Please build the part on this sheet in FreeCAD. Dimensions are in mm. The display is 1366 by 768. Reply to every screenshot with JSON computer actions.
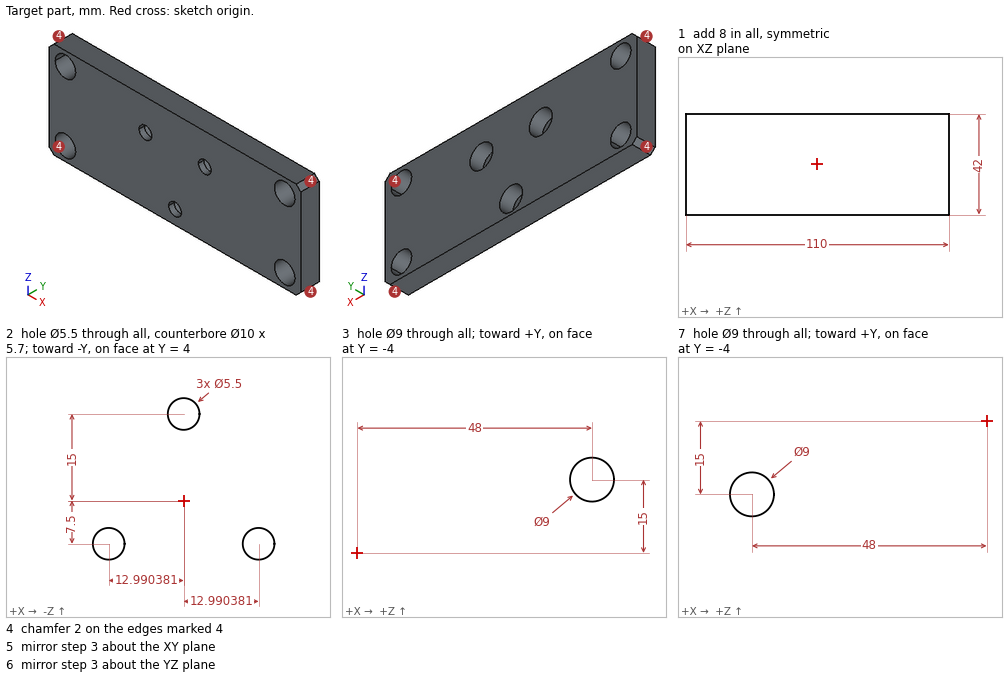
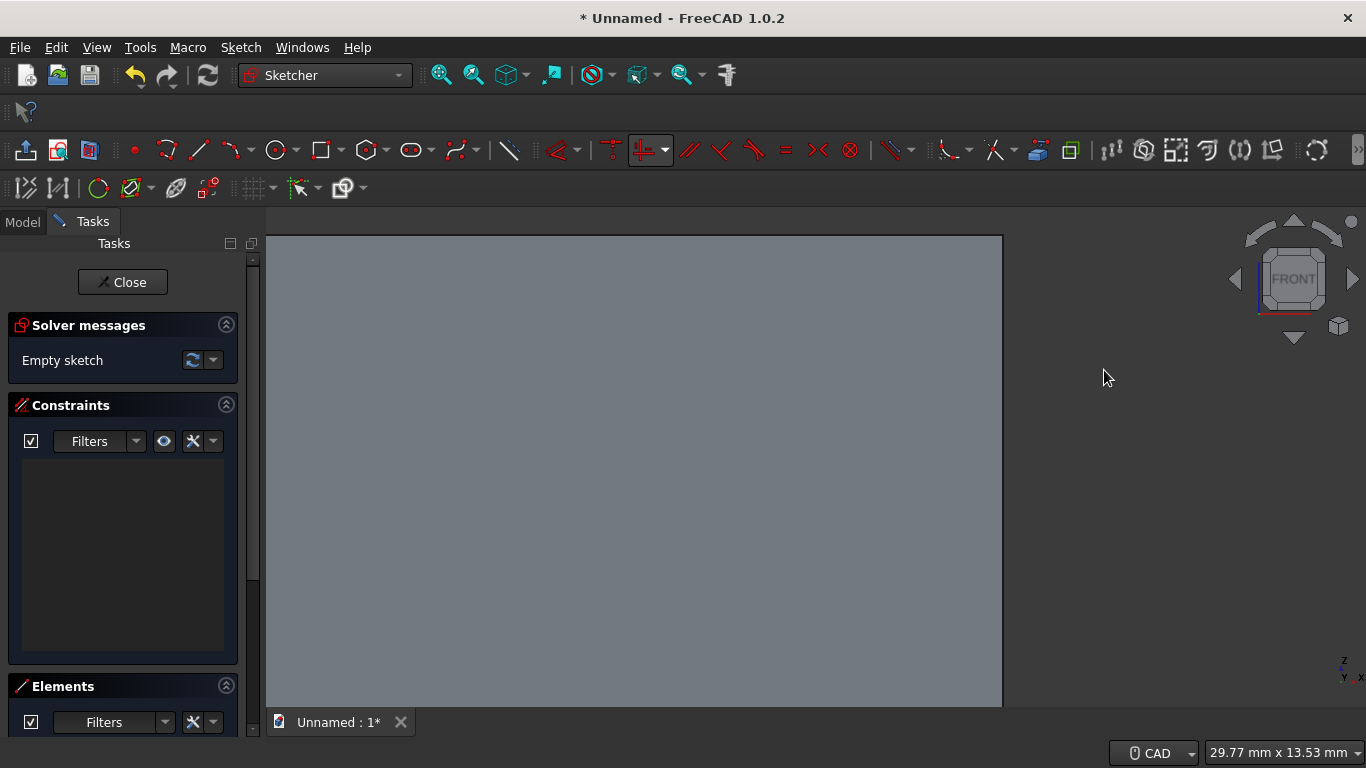
{"action": "left_click", "coordinate": [276, 150]}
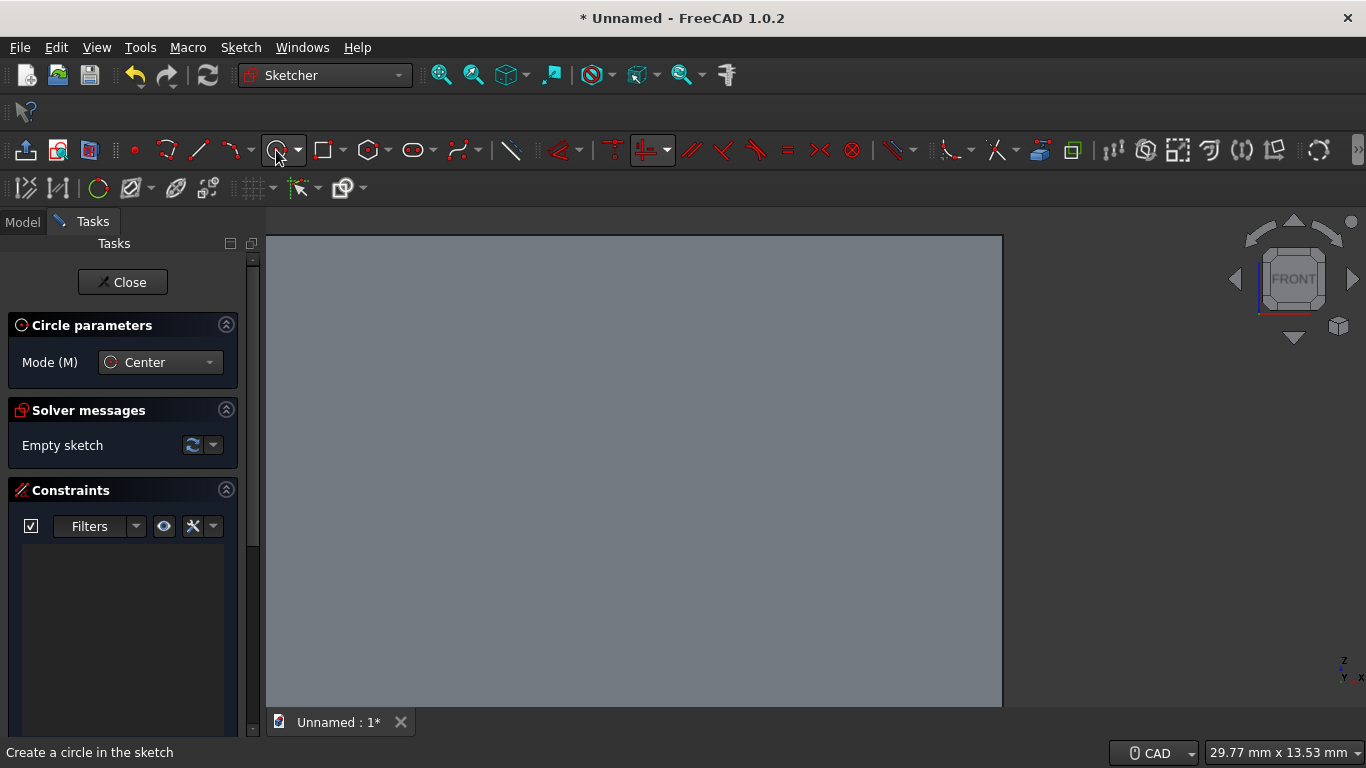
{"action": "left_click", "coordinate": [744, 457]}
{"action": "left_click", "coordinate": [862, 339]}
{"action": "key", "text": "Escape"}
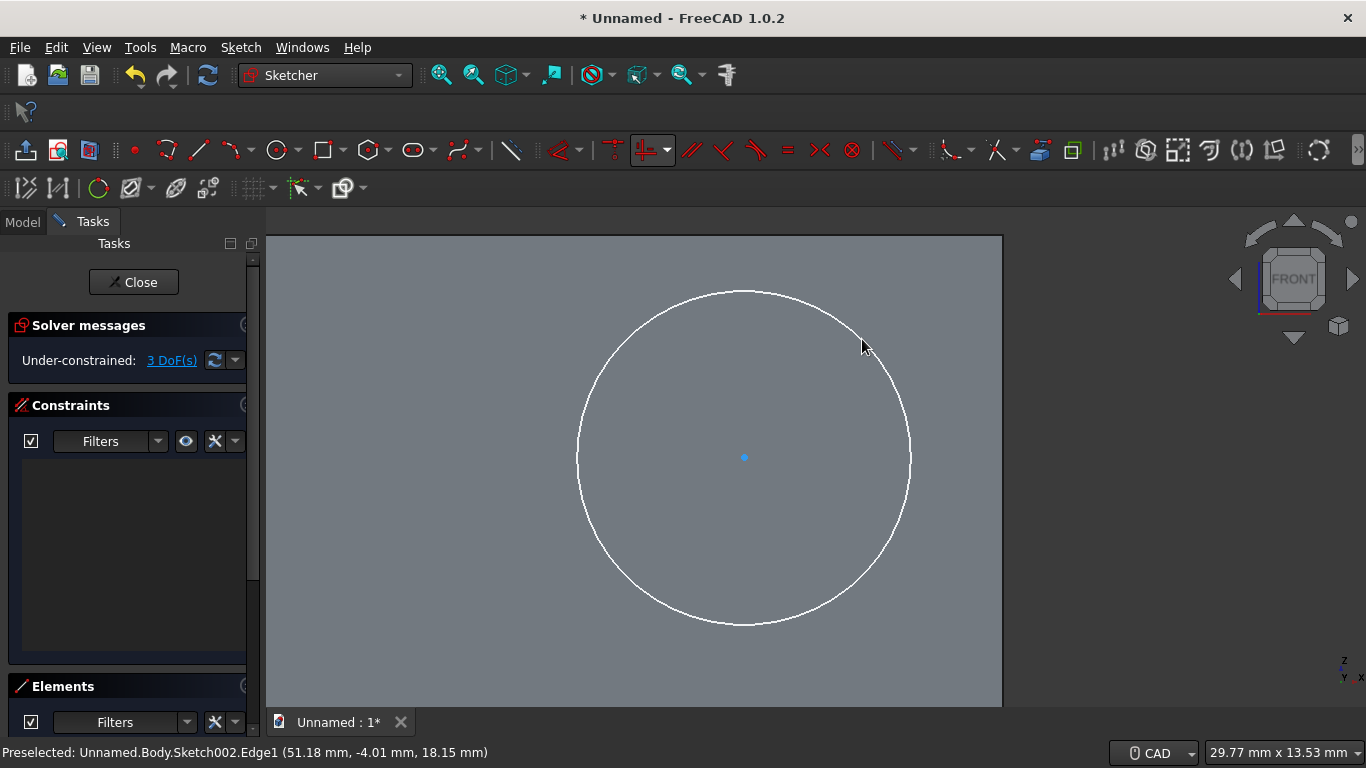
{"action": "left_click", "coordinate": [558, 150]}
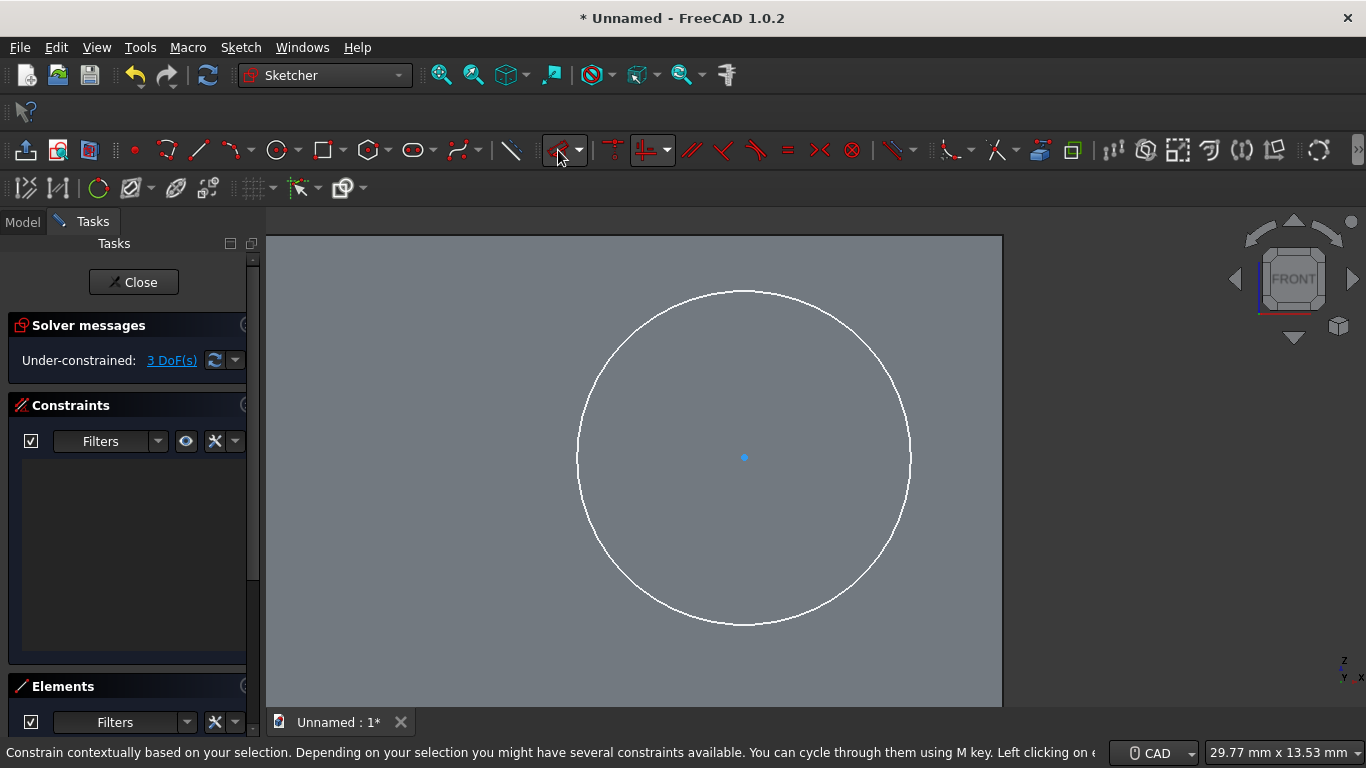
{"action": "left_click", "coordinate": [862, 340]}
{"action": "left_click", "coordinate": [885, 317]}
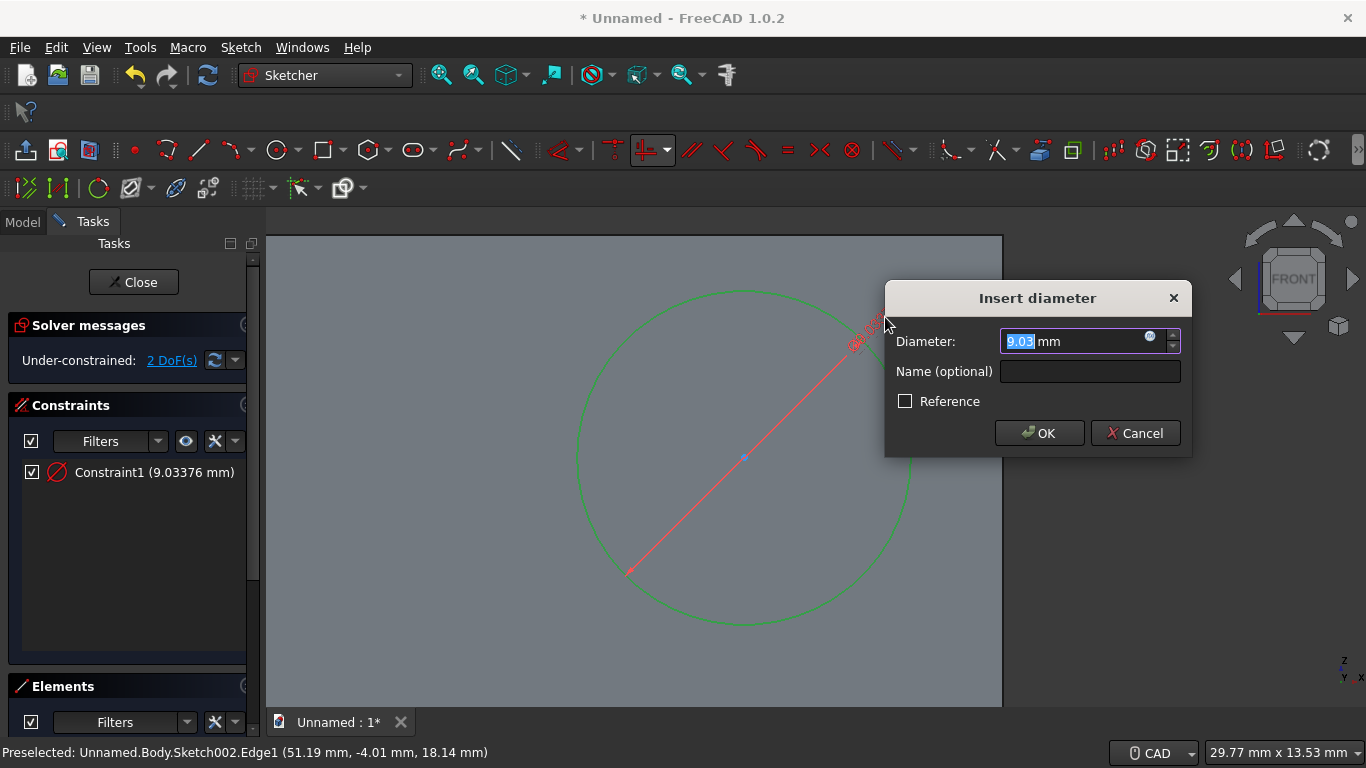
{"action": "type", "text": "9"}
{"action": "key", "text": "Return"}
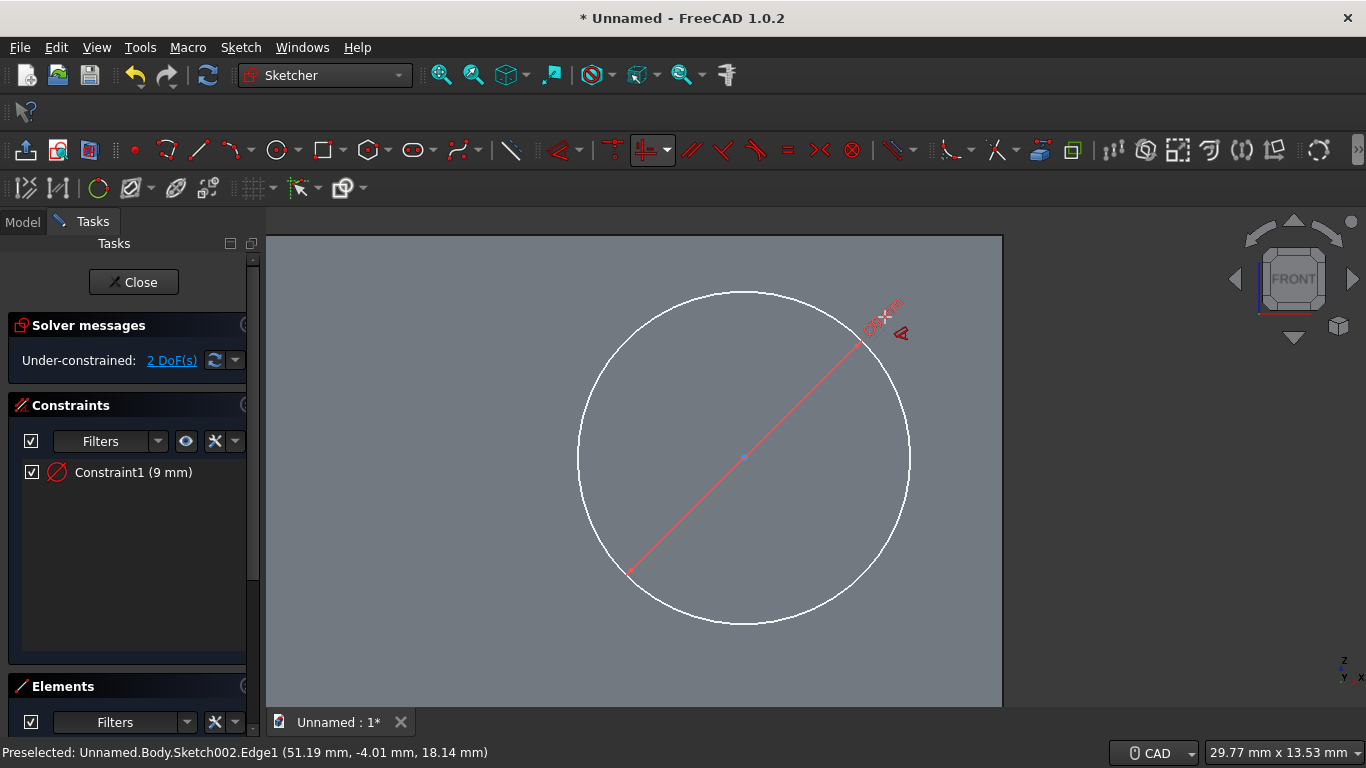
{"action": "left_click", "coordinate": [744, 458]}
{"action": "left_click", "coordinate": [519, 424]}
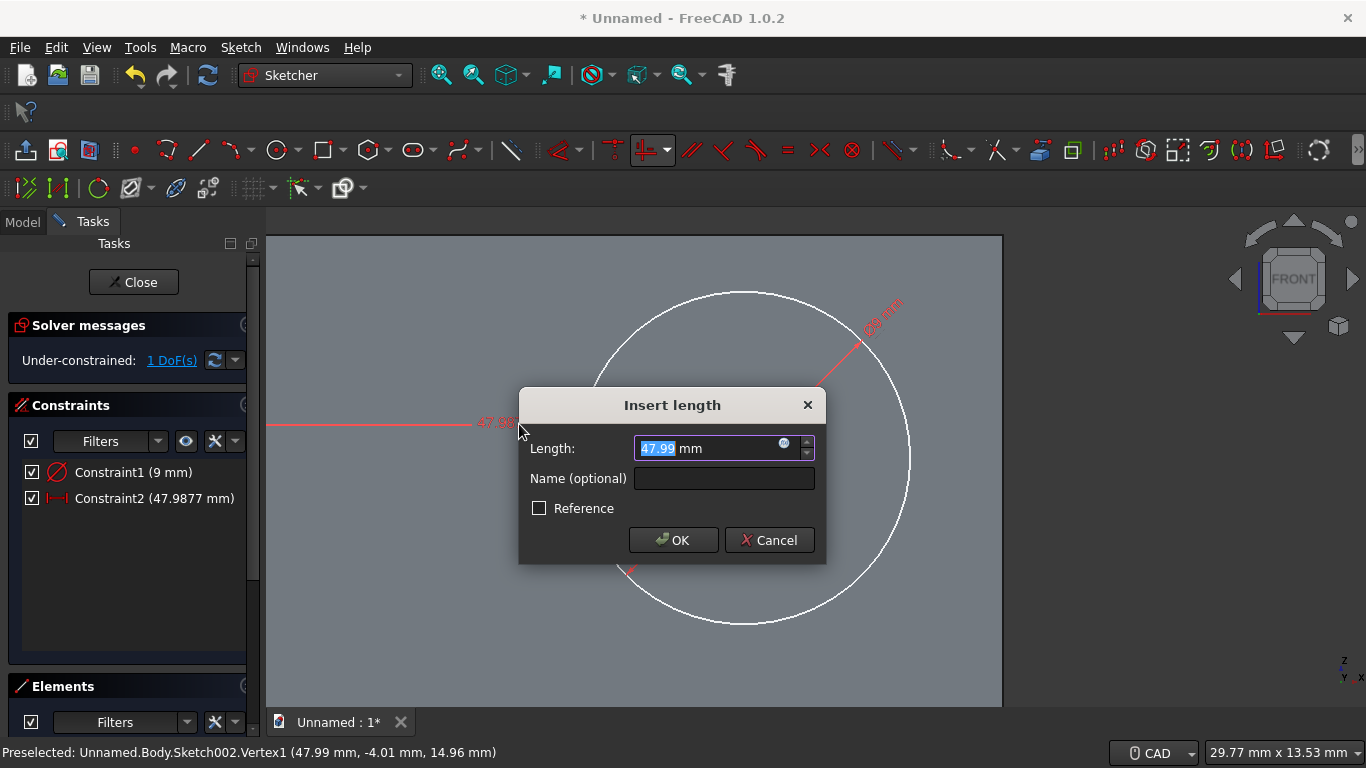
{"action": "type", "text": "48"}
{"action": "key", "text": "Return"}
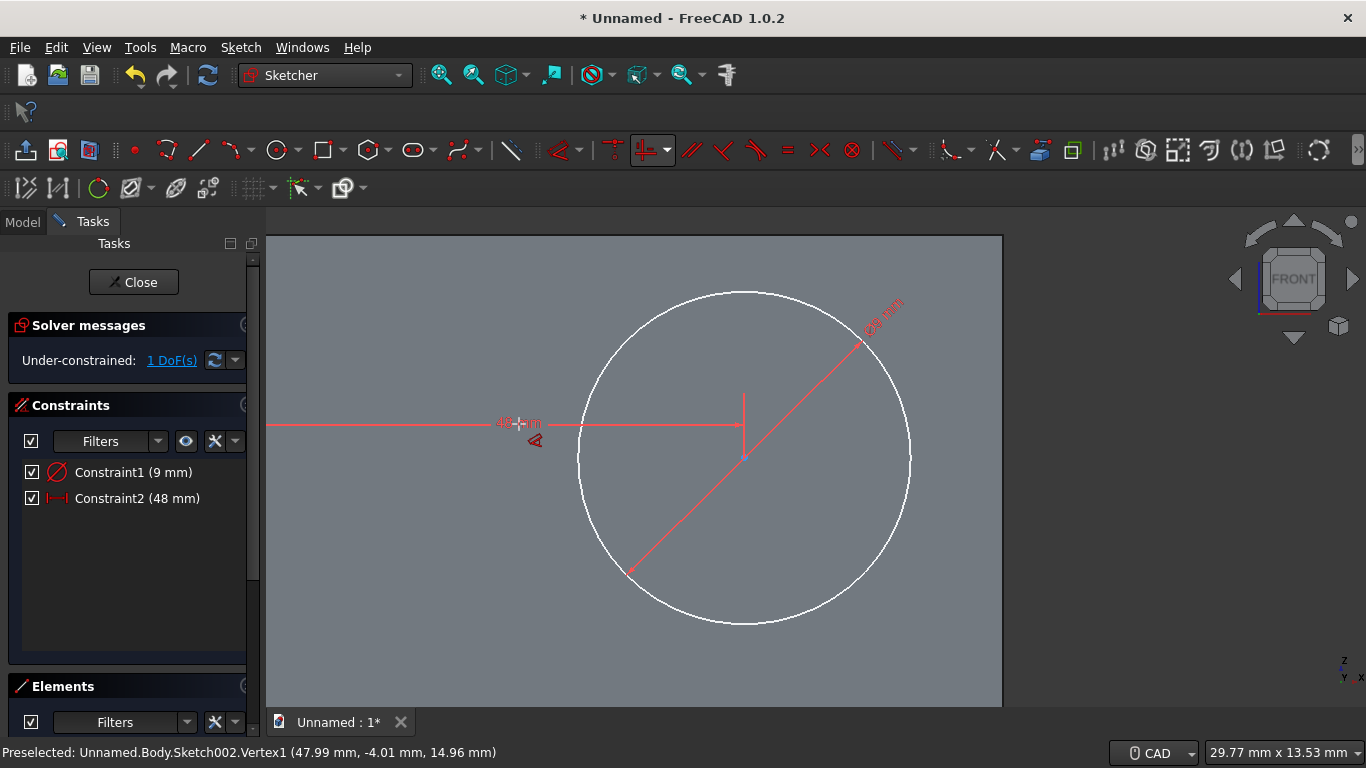
{"action": "left_click", "coordinate": [744, 458]}
{"action": "left_click", "coordinate": [778, 568]}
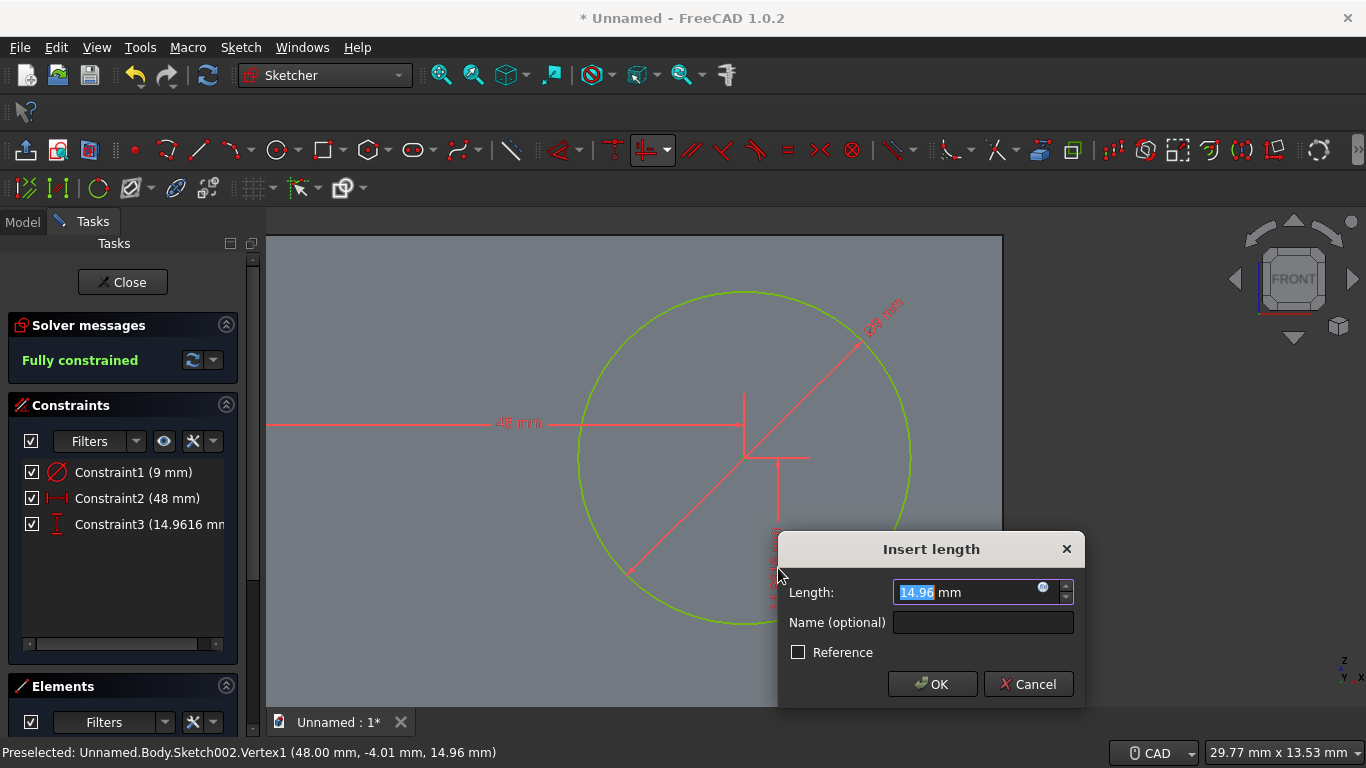
{"action": "type", "text": "15"}
{"action": "key", "text": "Return"}
{"action": "key", "text": "Escape"}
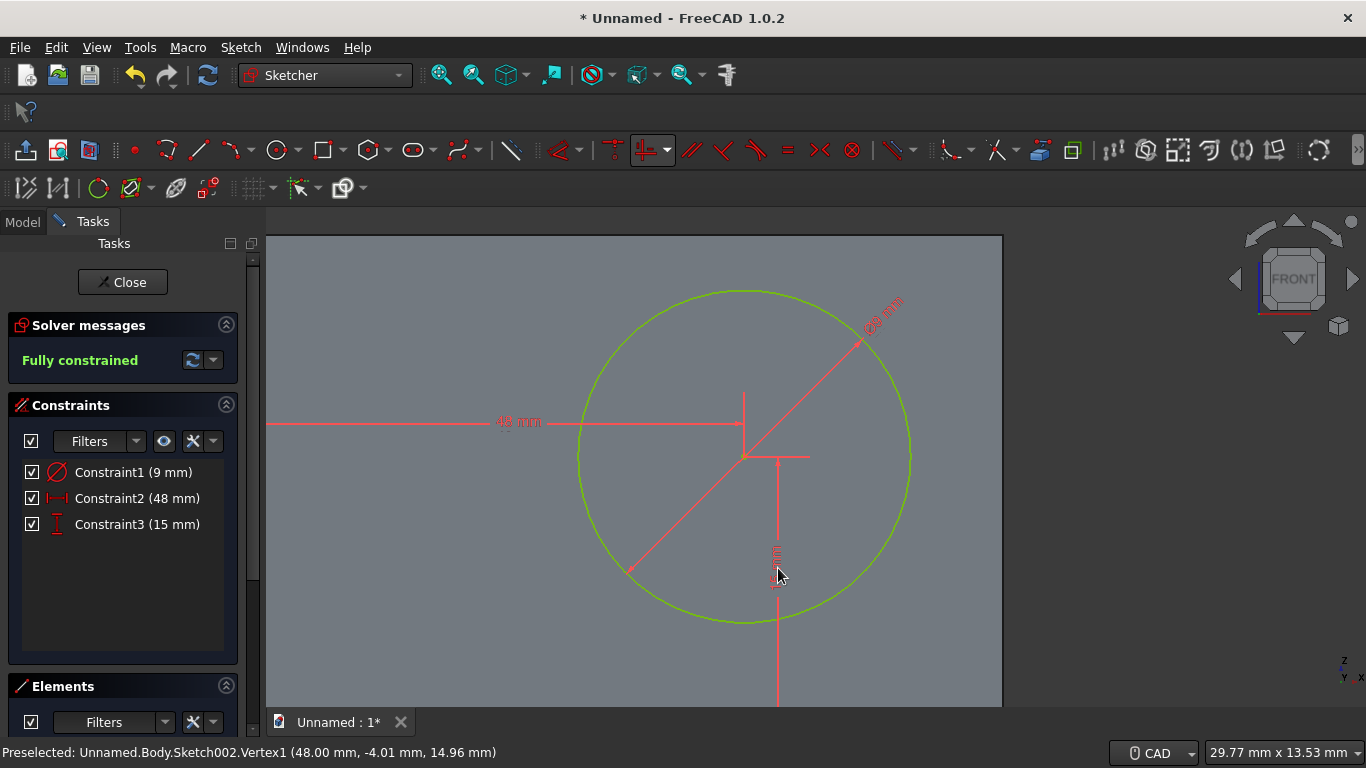
{"action": "left_click", "coordinate": [123, 282]}